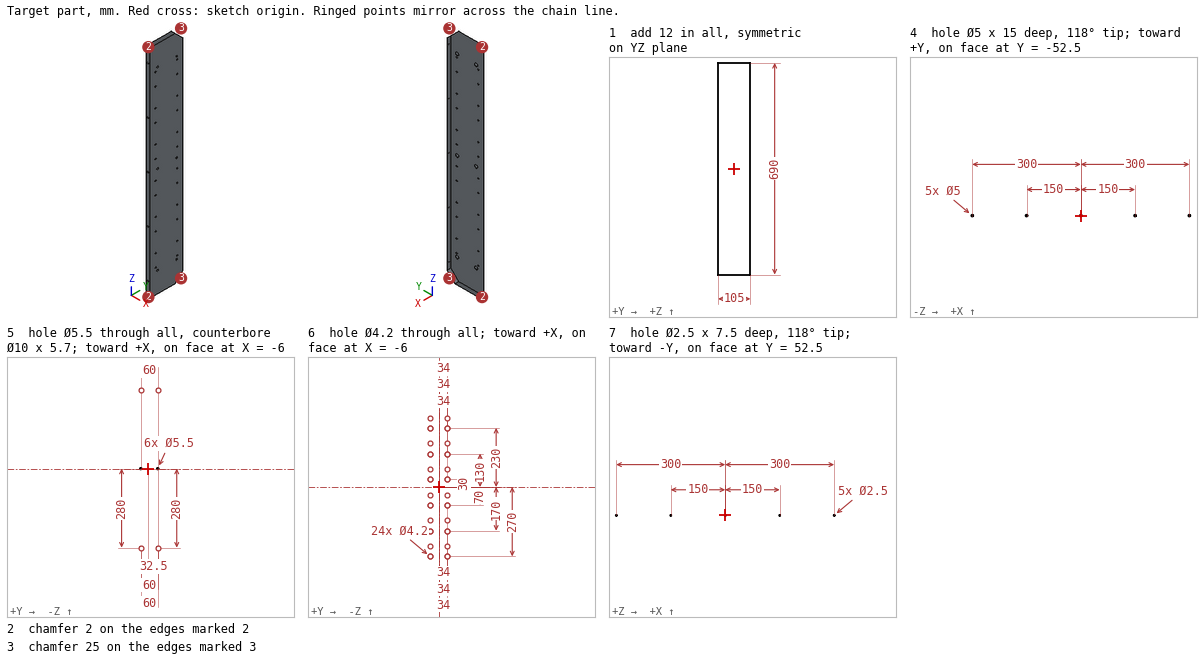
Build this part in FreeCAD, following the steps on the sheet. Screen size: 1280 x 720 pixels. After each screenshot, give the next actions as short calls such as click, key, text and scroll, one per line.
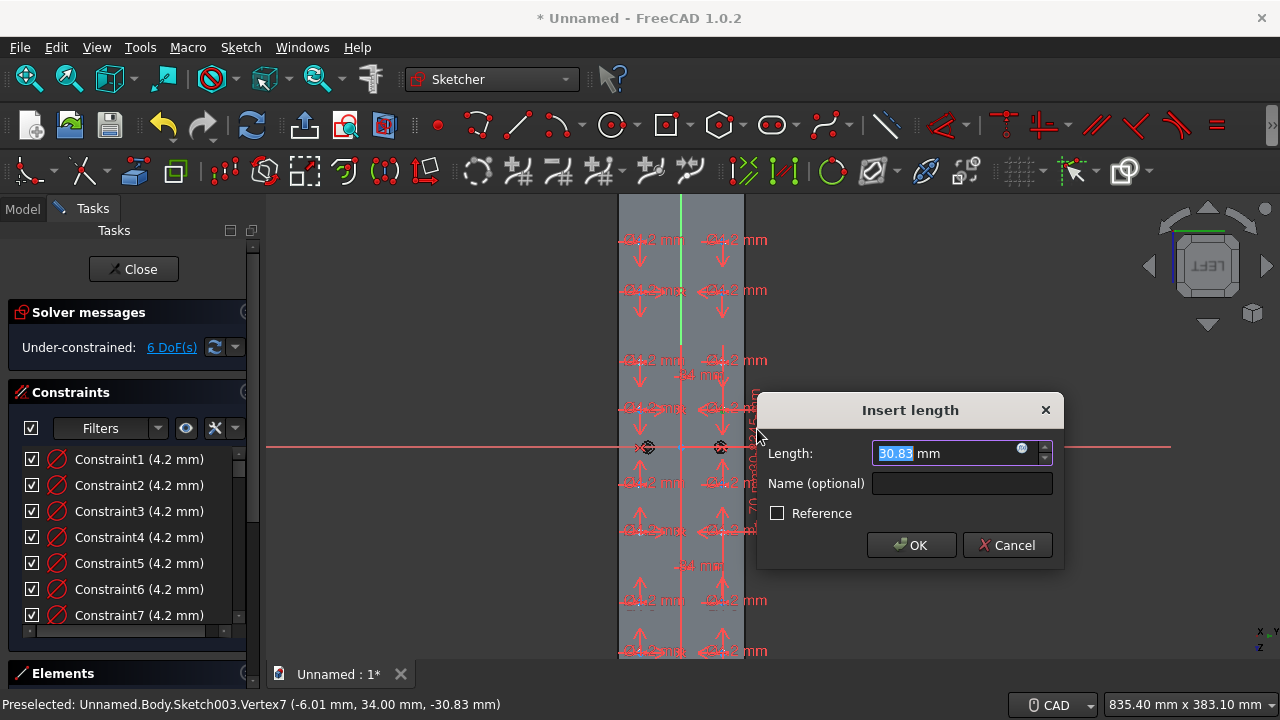
text(30)
key(Return)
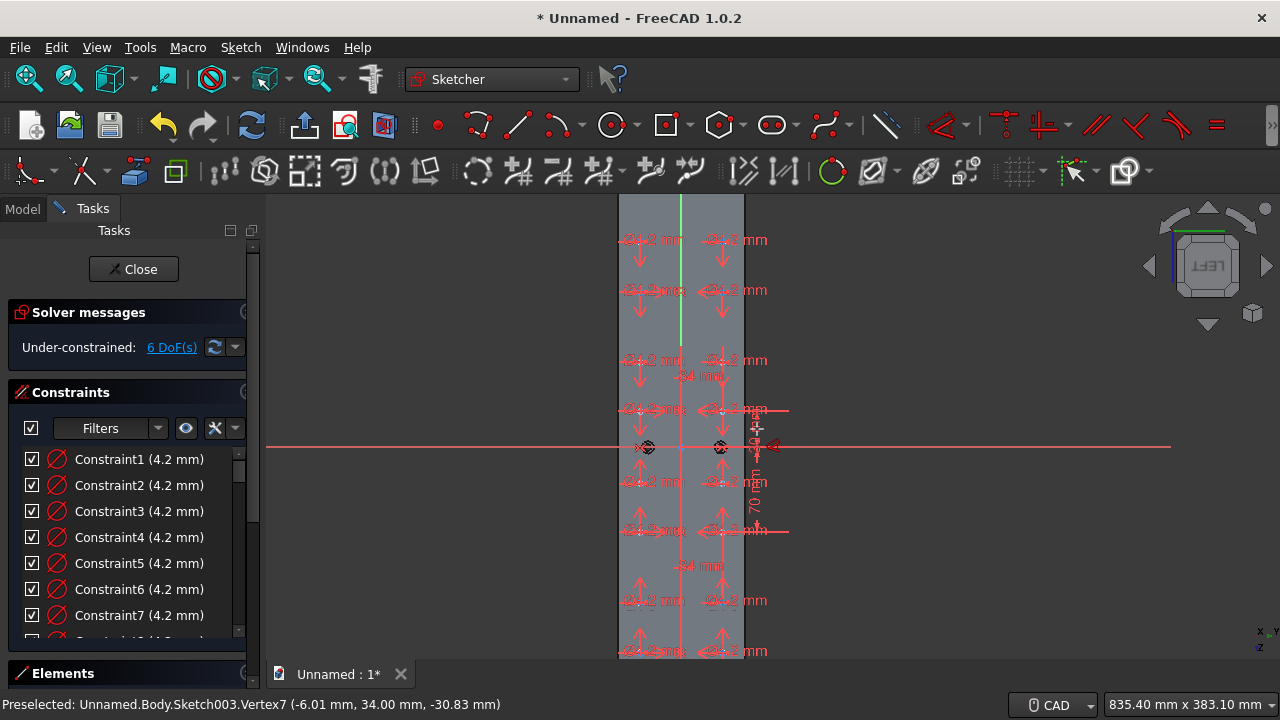
click(722, 292)
click(702, 258)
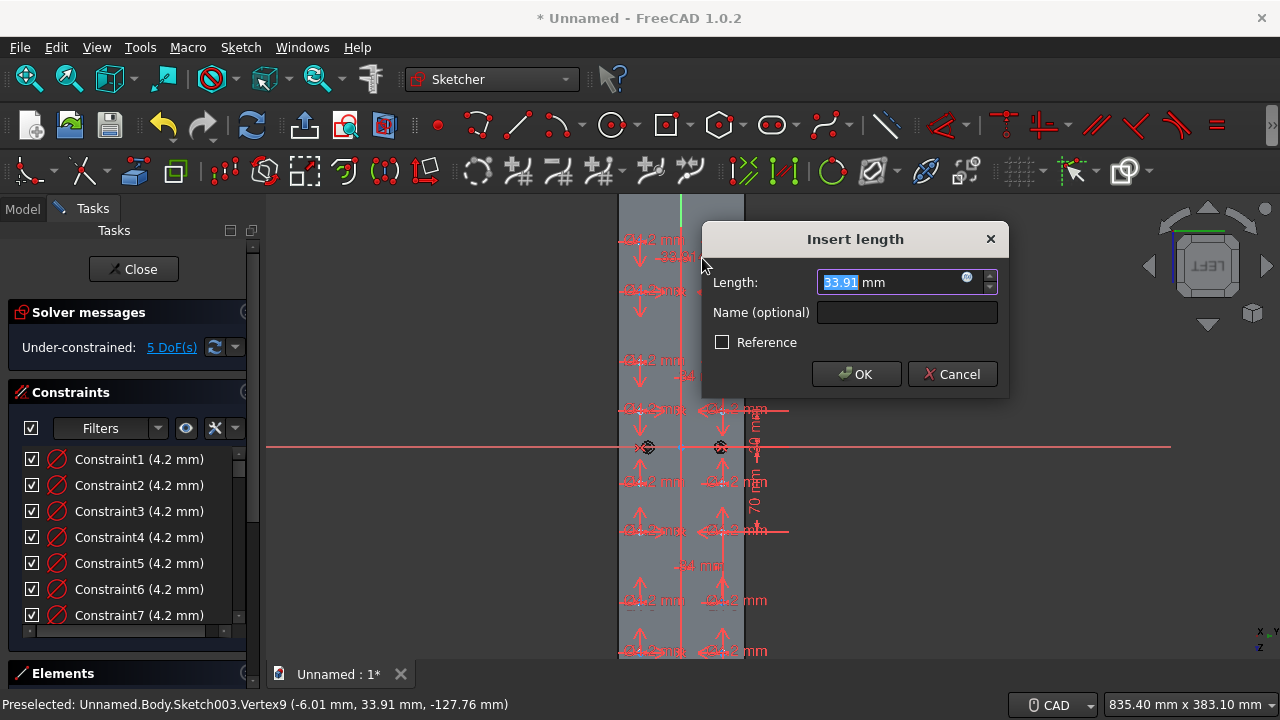
text(34)
key(Return)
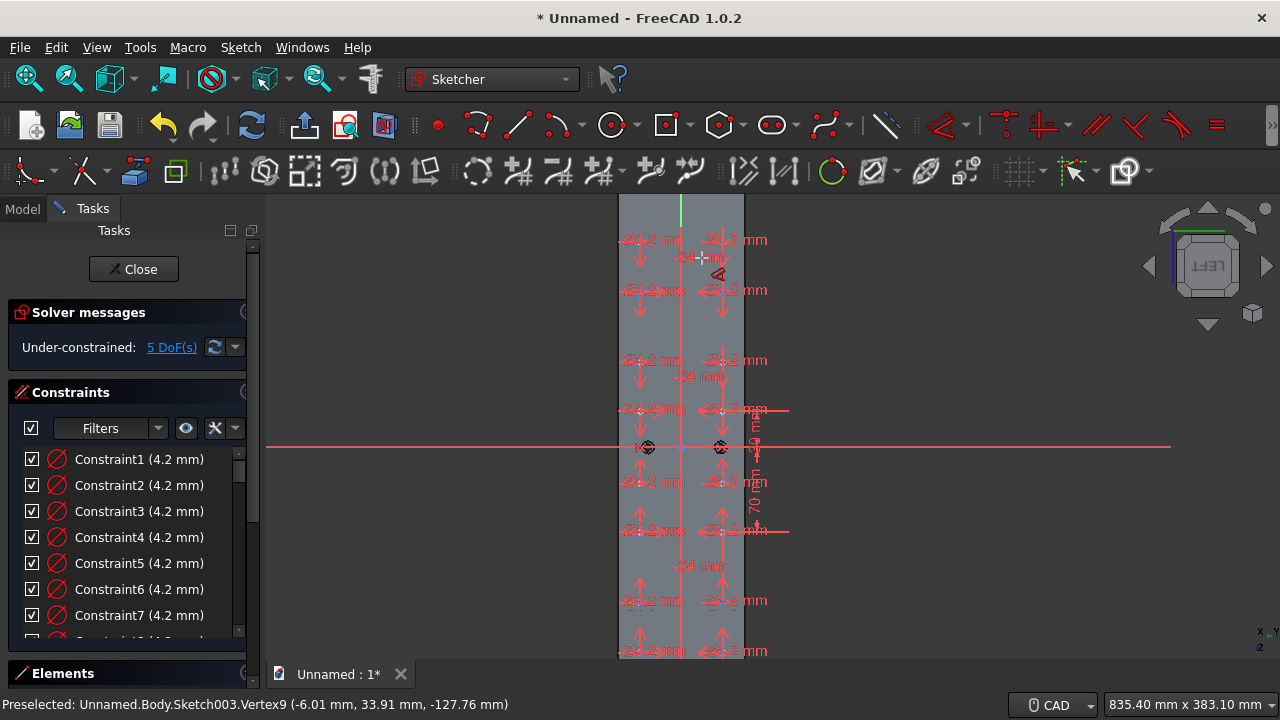
scroll(723, 409, down, 4)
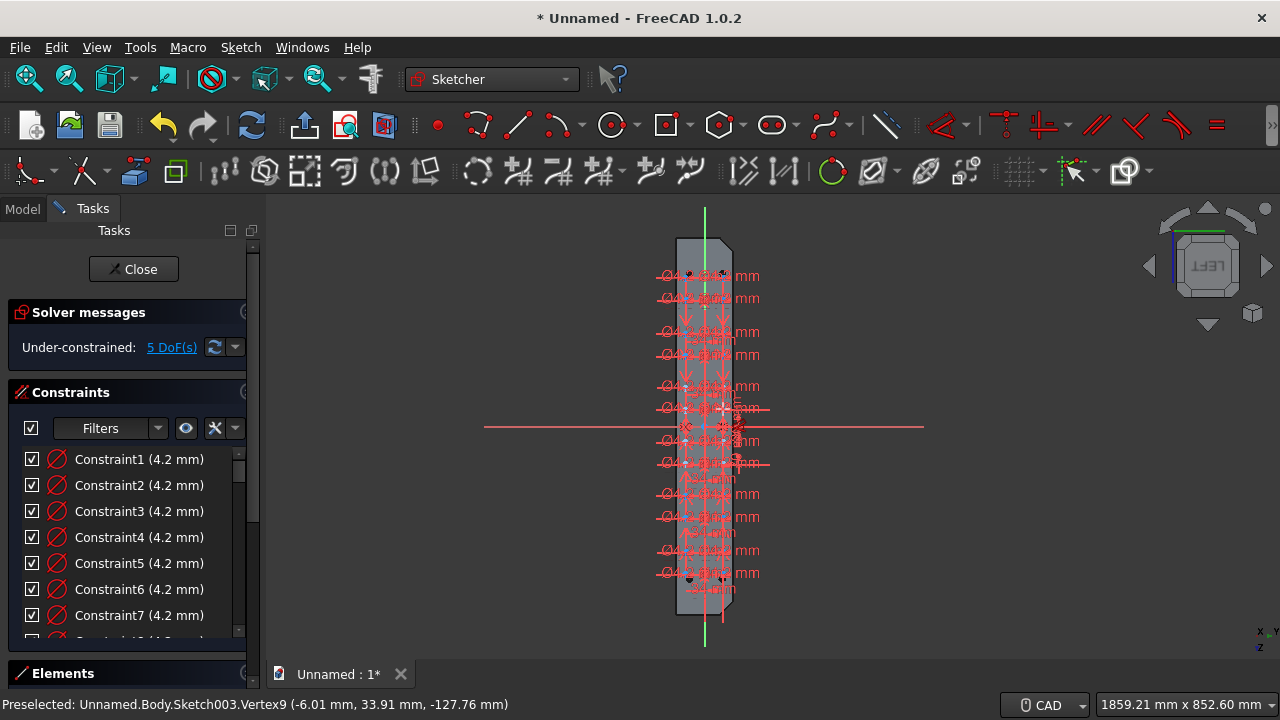
scroll(723, 301, up, 4)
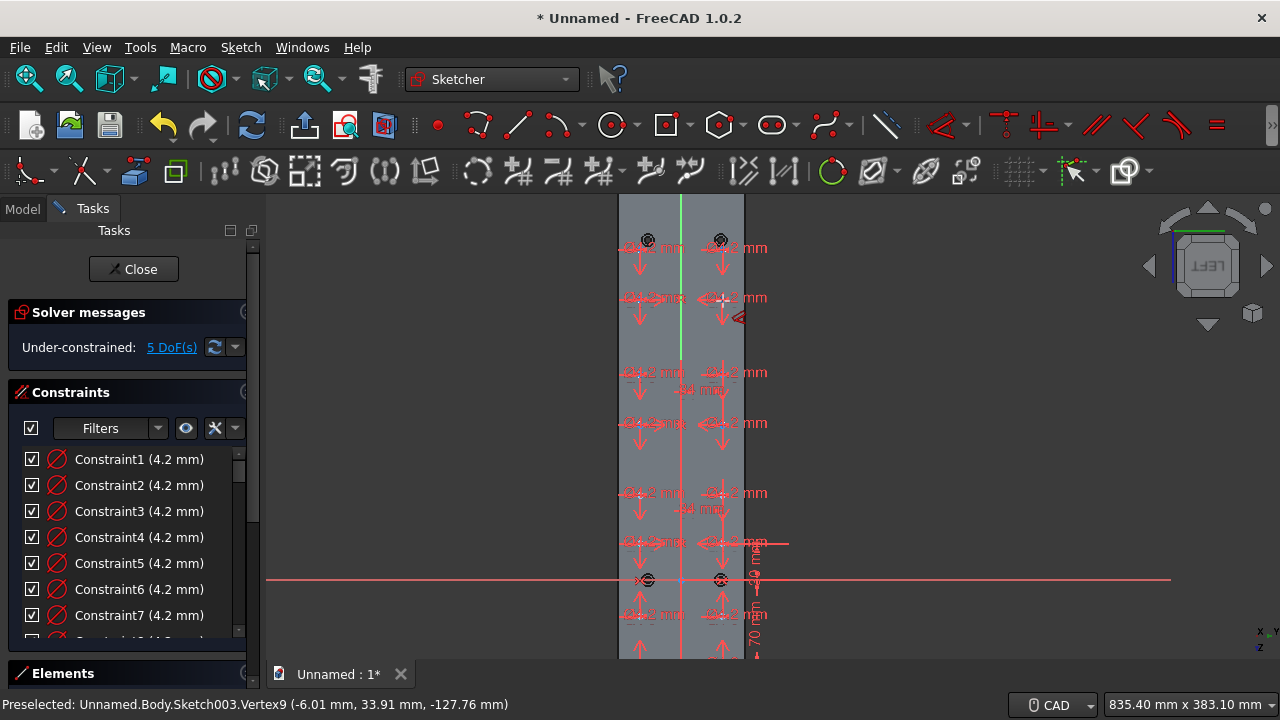
click(722, 300)
click(702, 266)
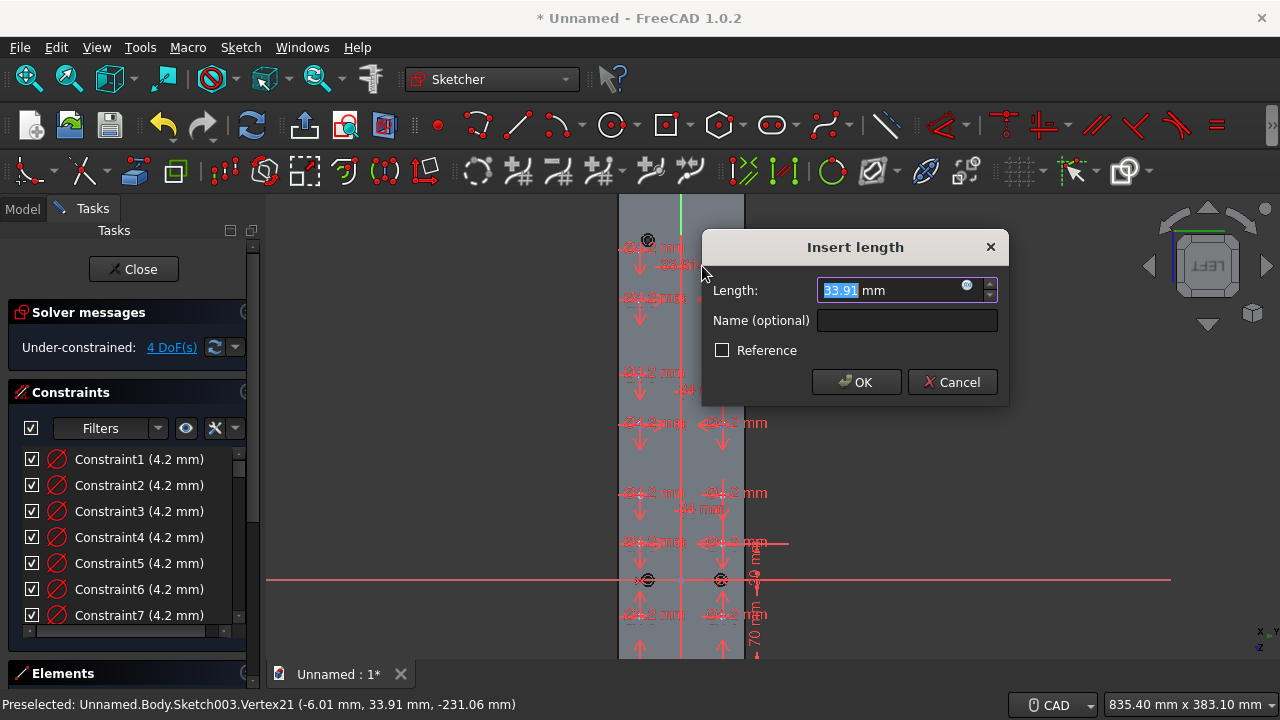
text(34)
key(Return)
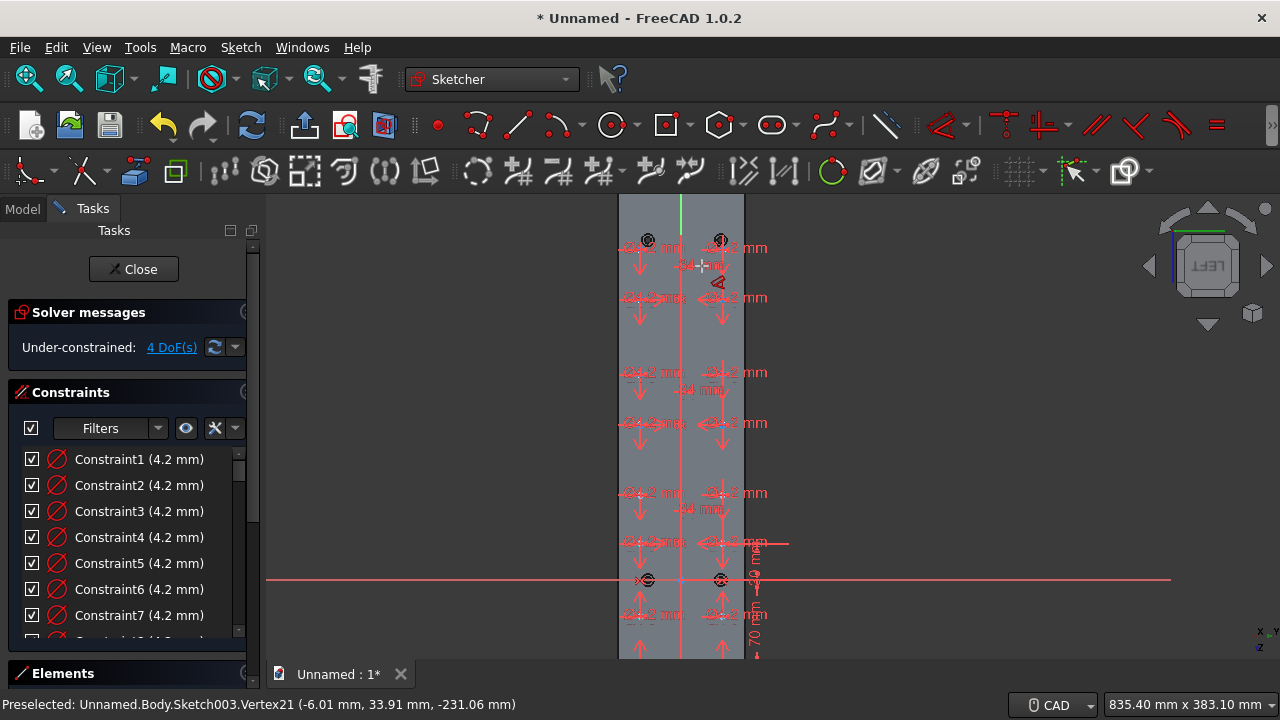
scroll(723, 301, down, 4)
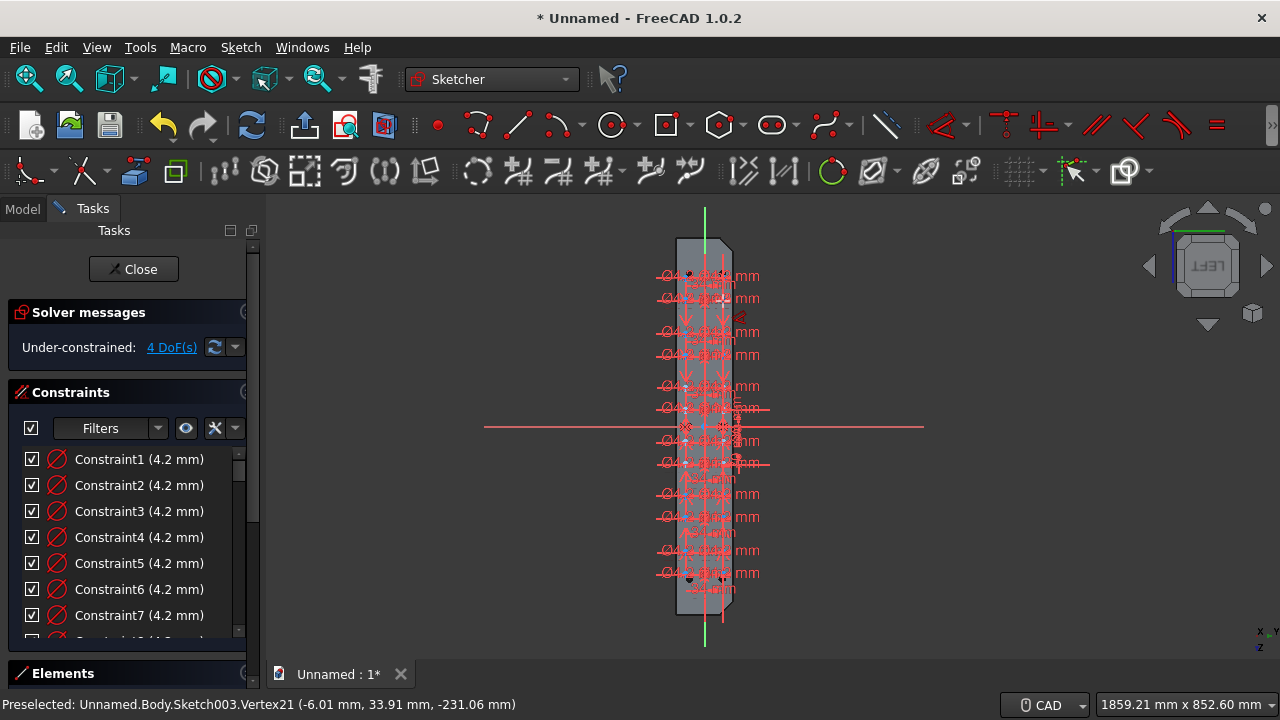
click(723, 575)
click(757, 501)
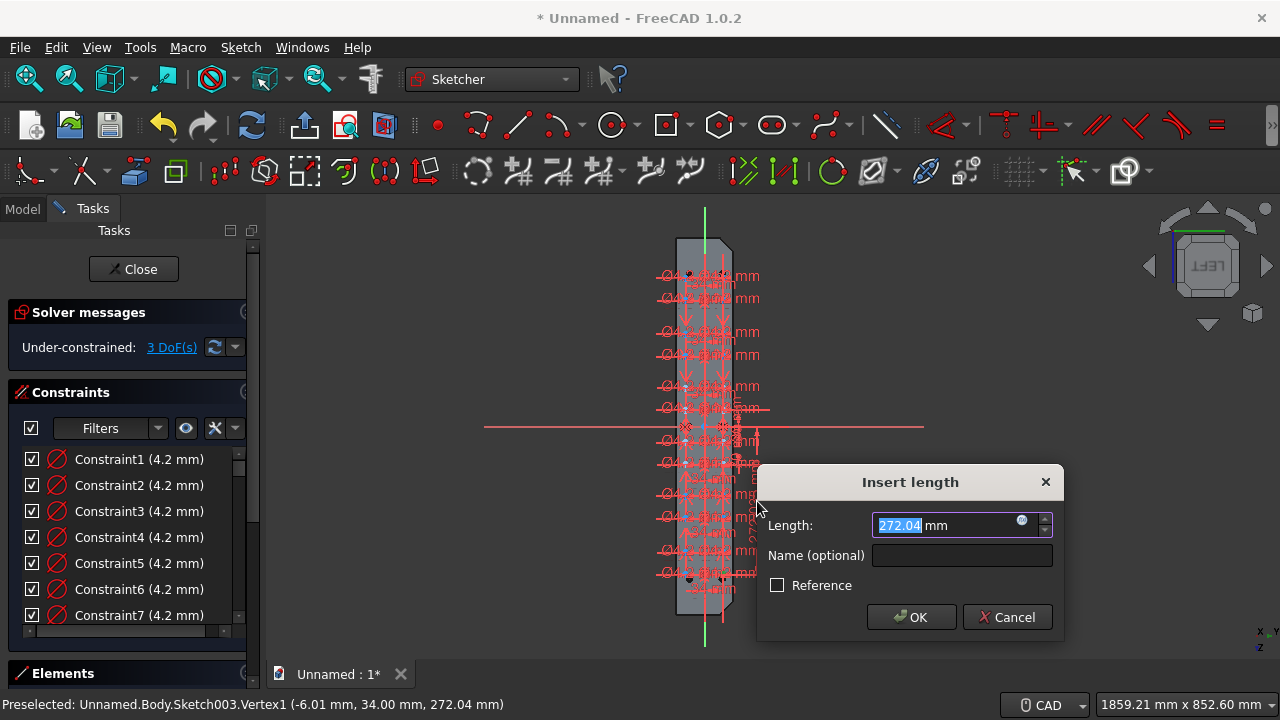
text(270)
key(Return)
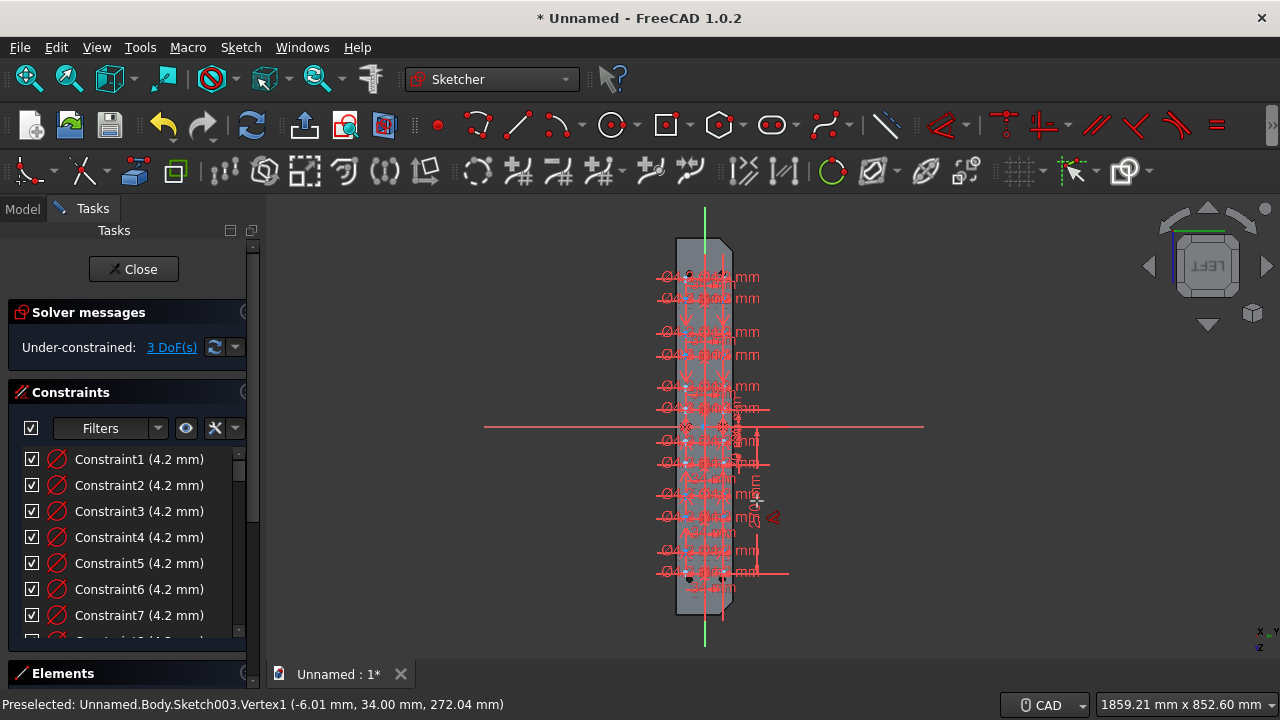
click(723, 519)
click(671, 505)